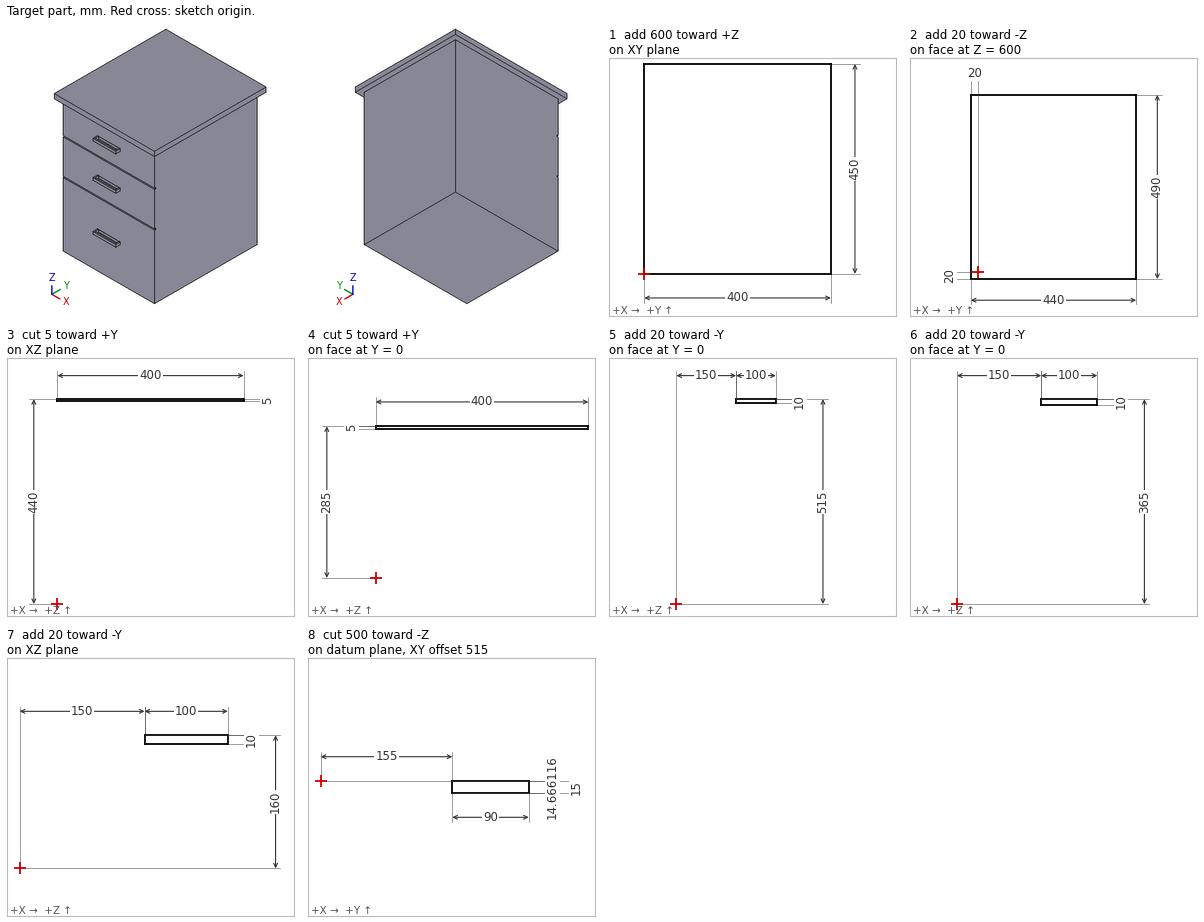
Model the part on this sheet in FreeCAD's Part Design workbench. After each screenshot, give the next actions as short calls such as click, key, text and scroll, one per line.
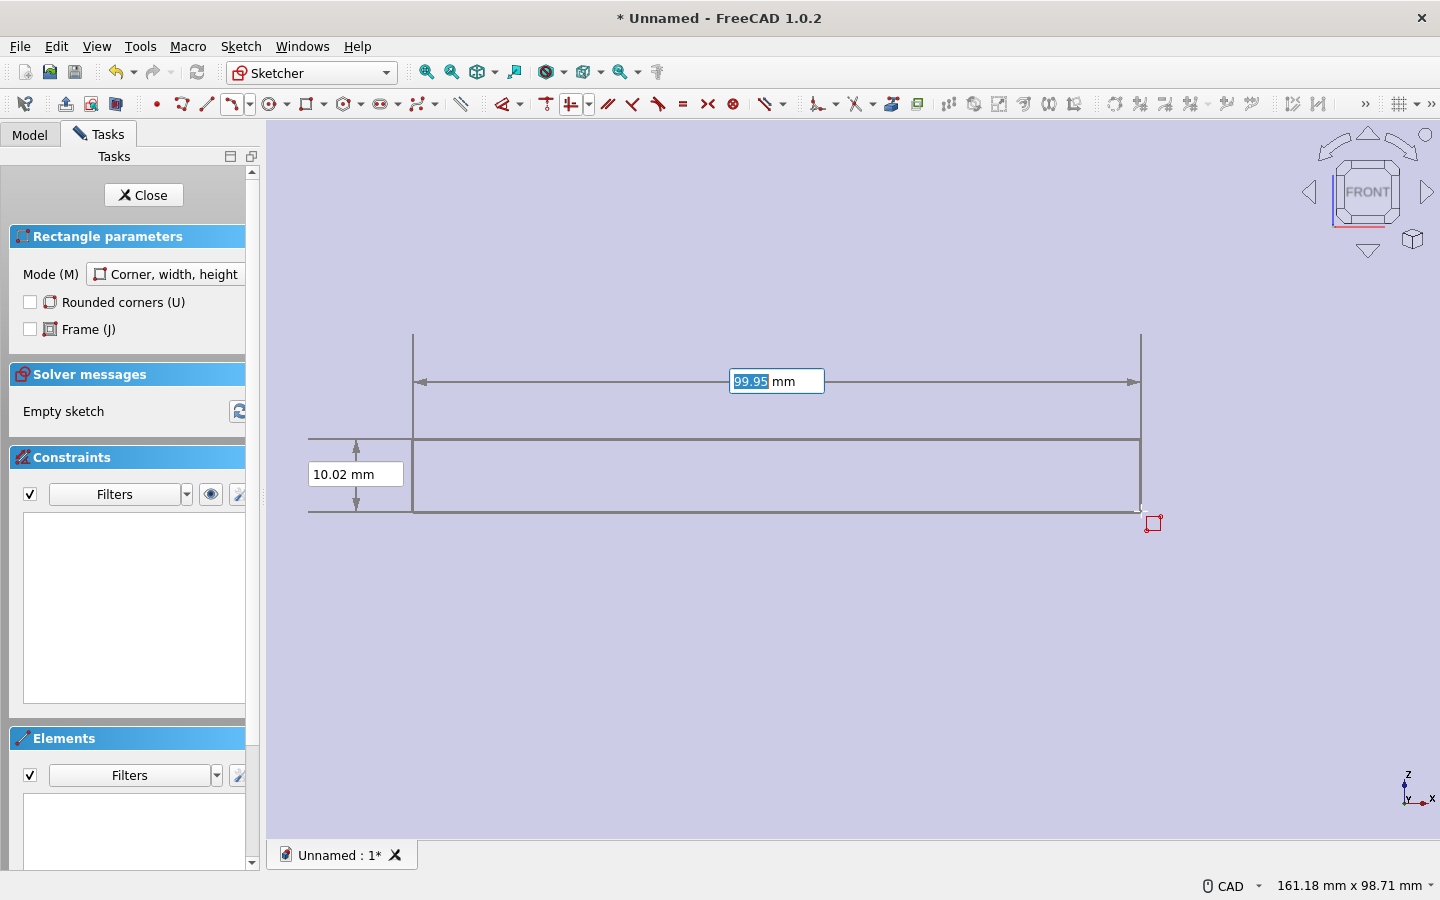
text(100)
key(Tab)
text(10)
key(Return)
key(Escape)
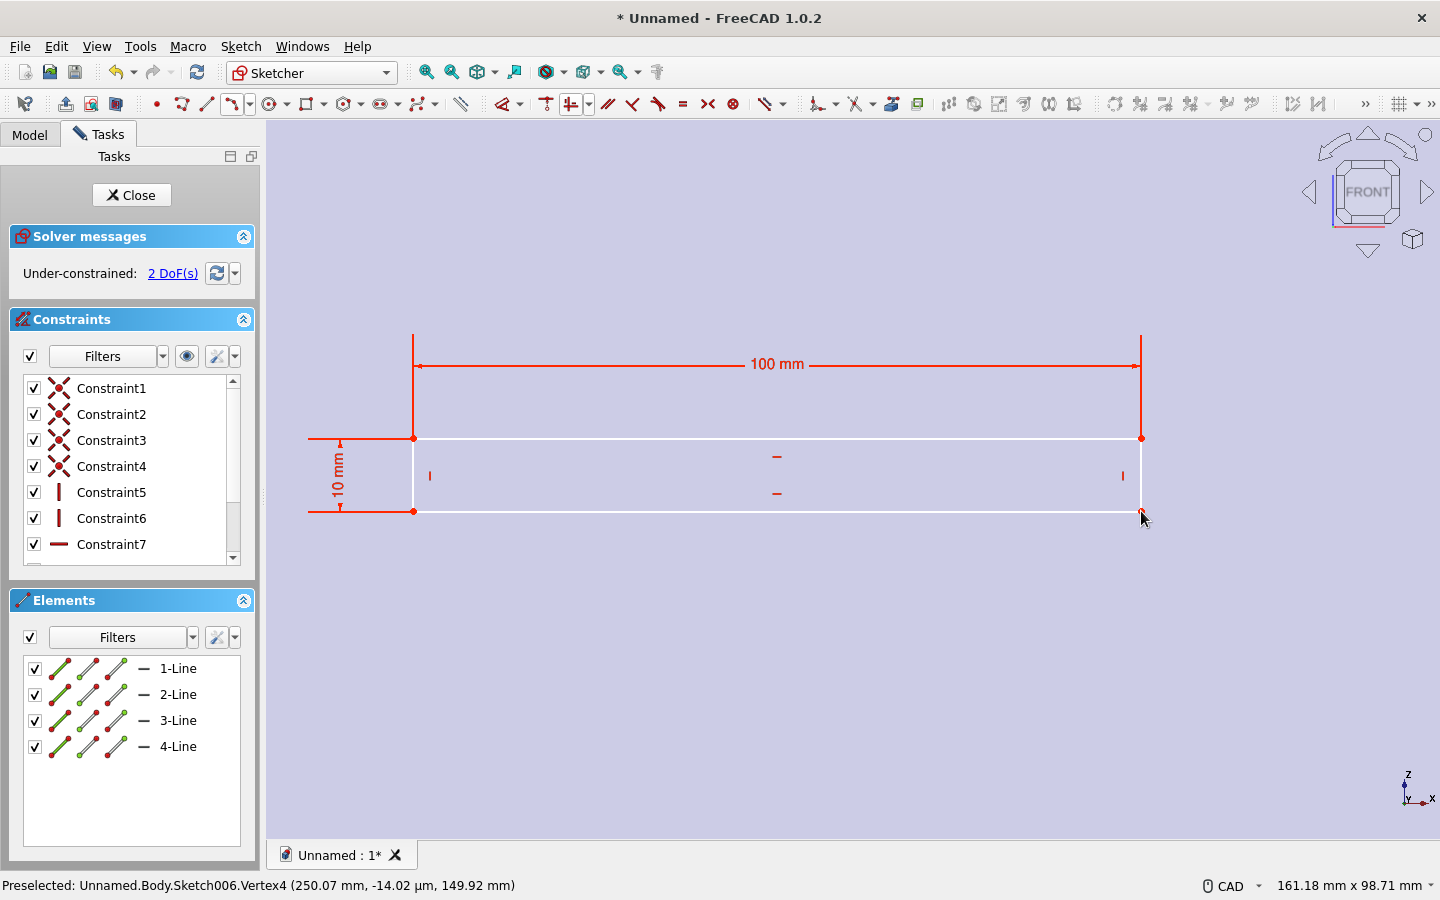
key(d)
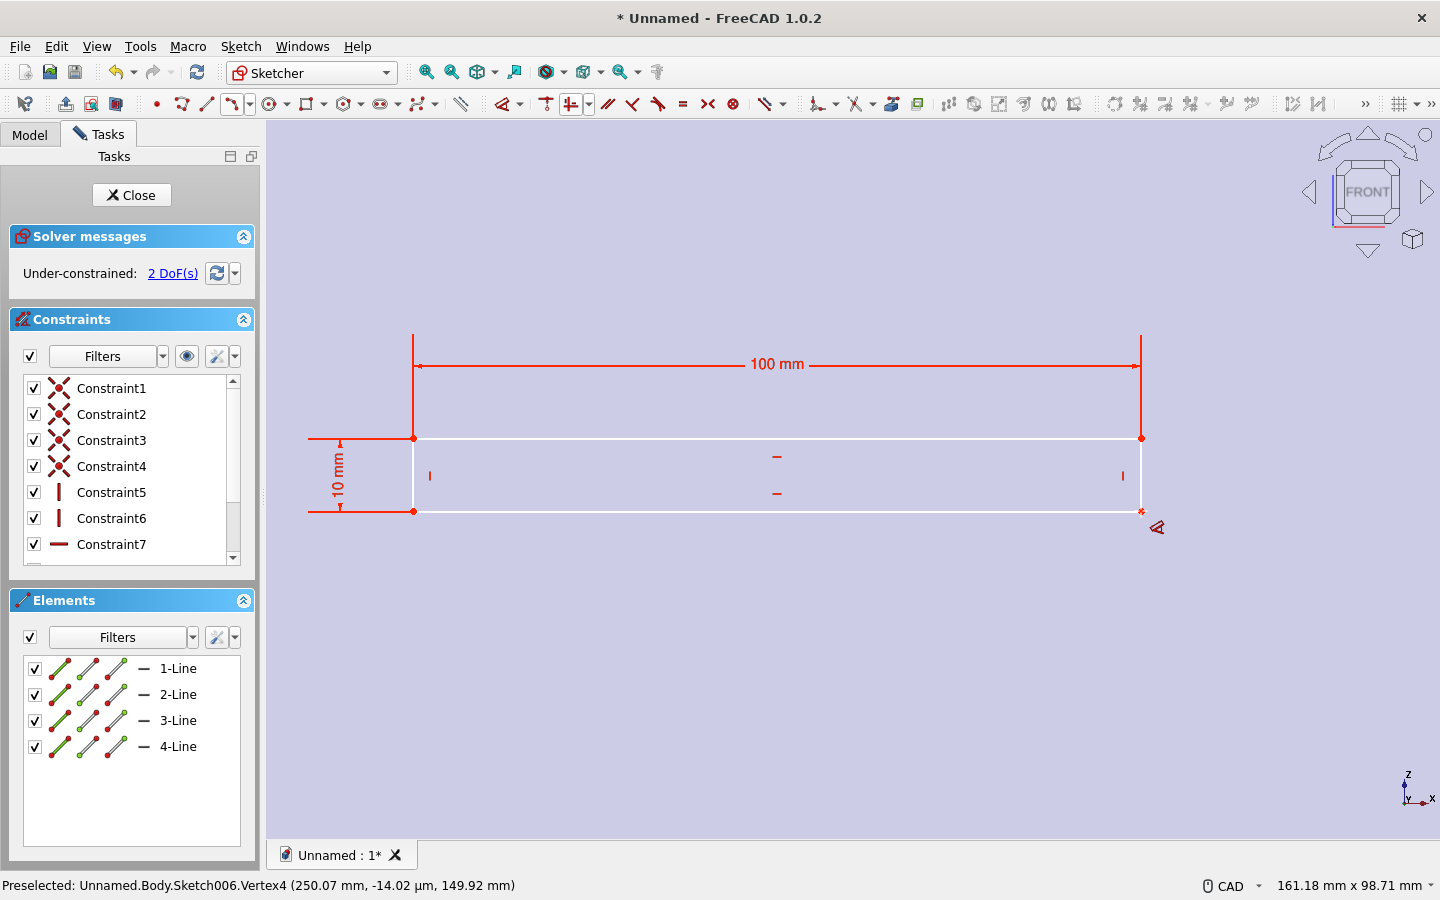
click(413, 439)
click(354, 405)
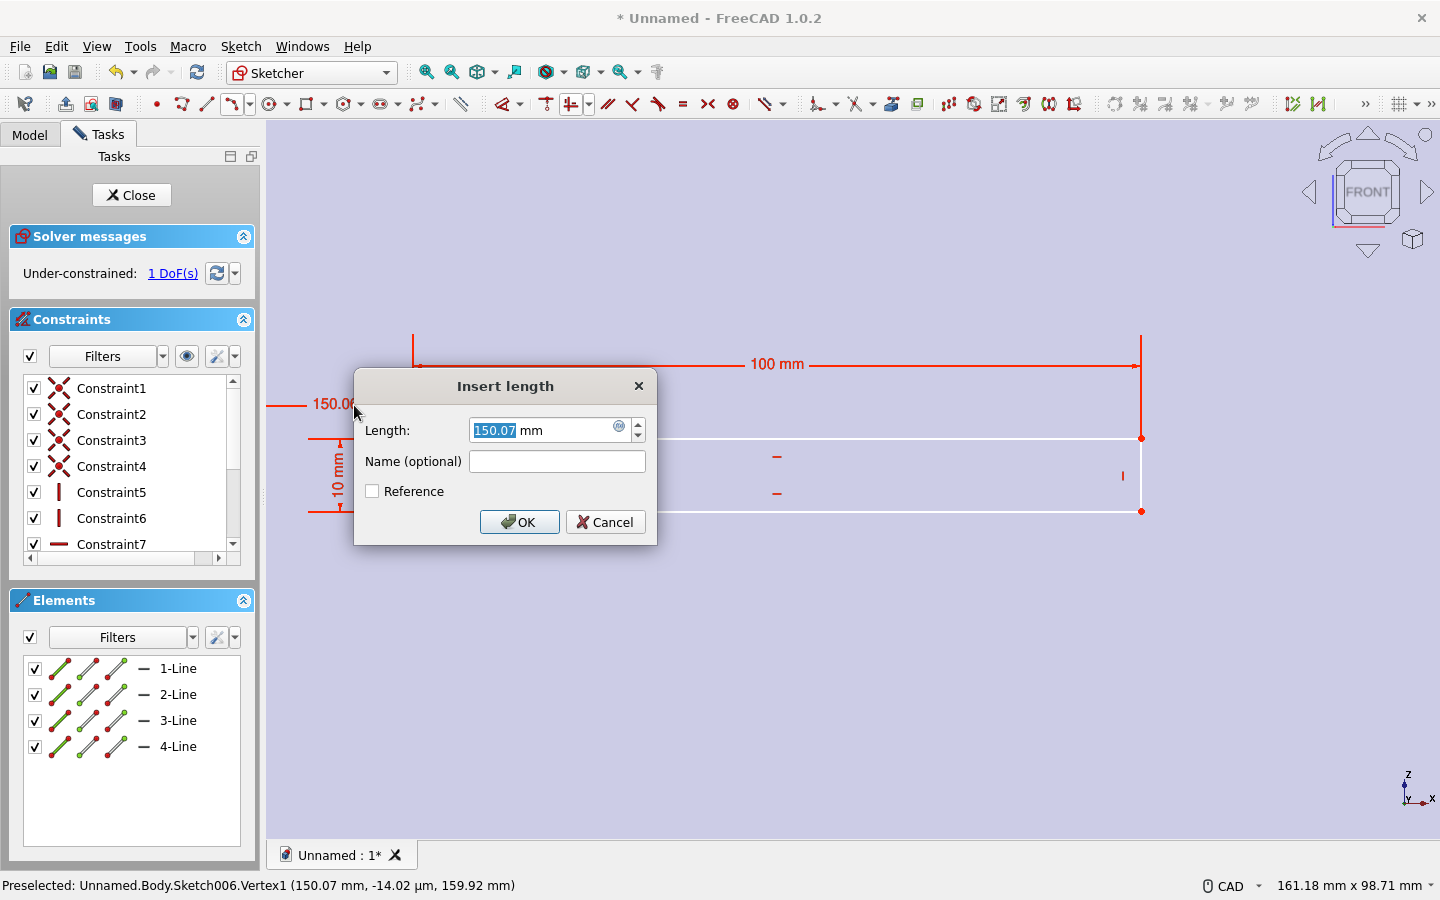
text(150)
key(Return)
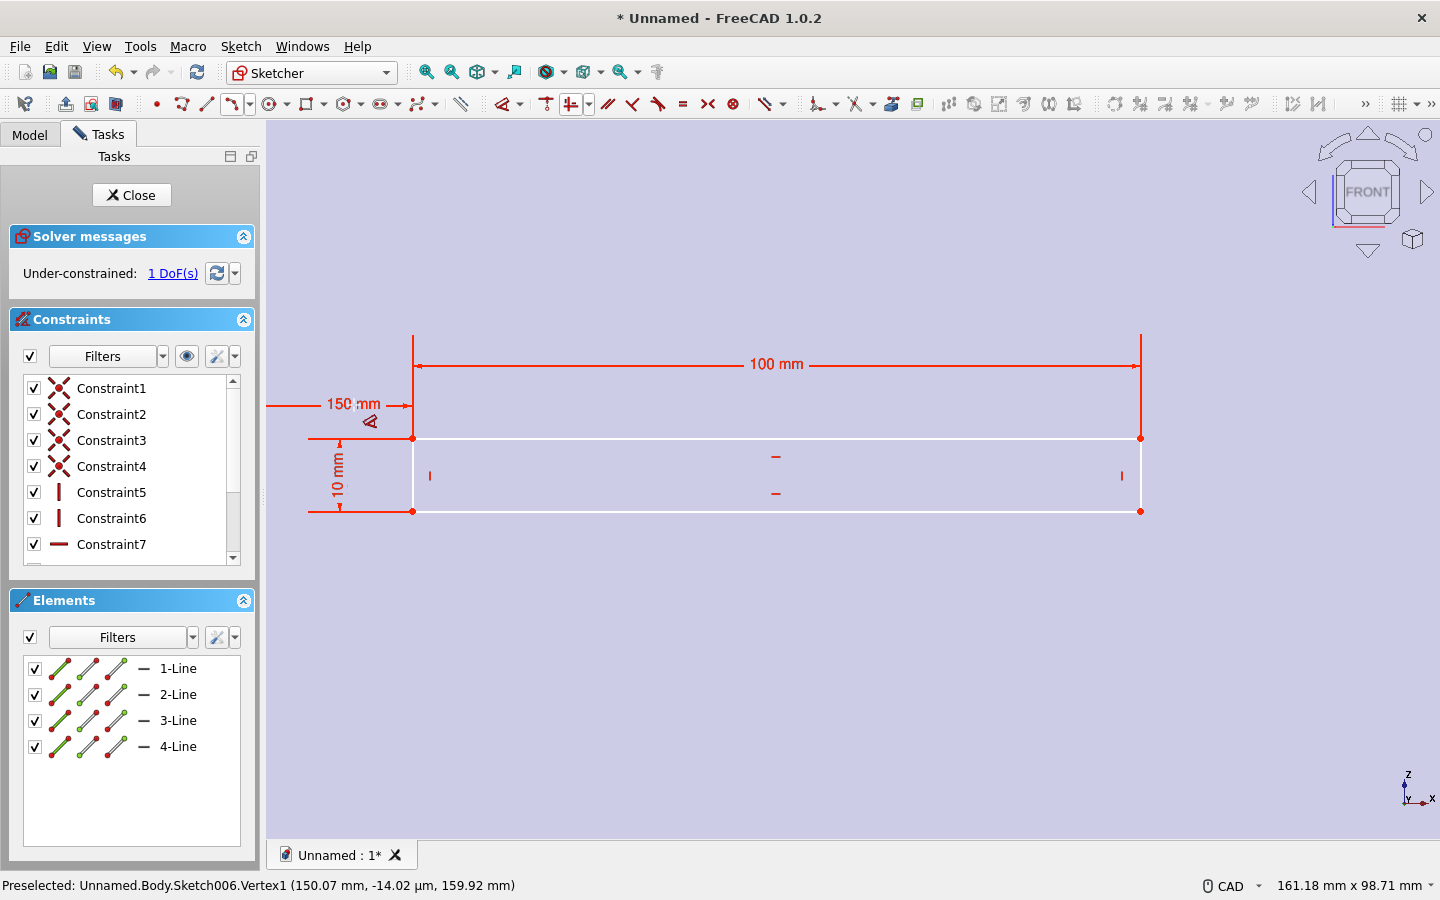
click(413, 439)
click(447, 625)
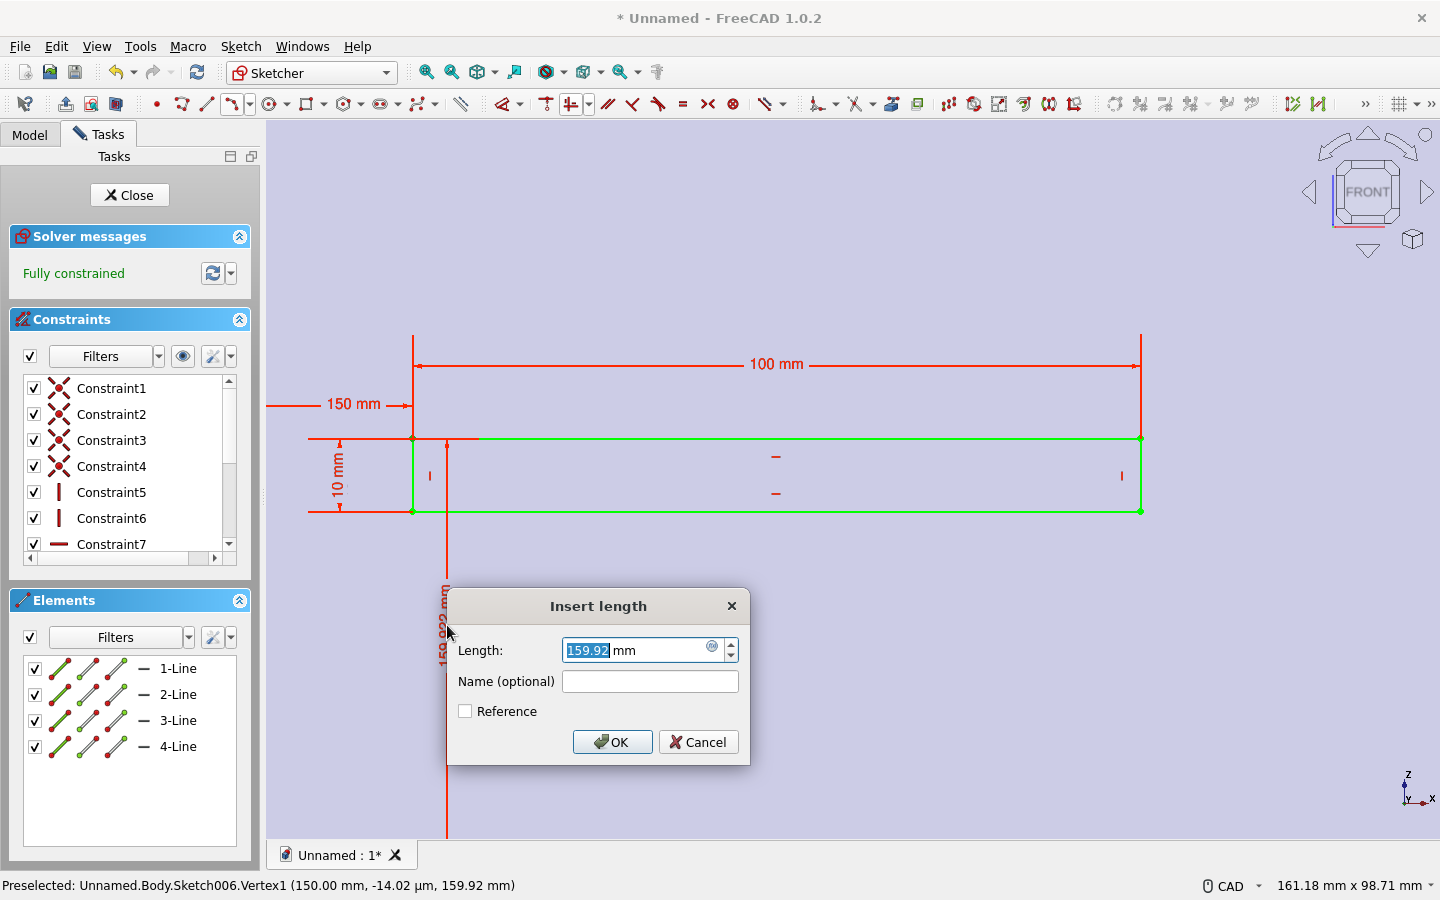
text(160)
key(Return)
key(Escape)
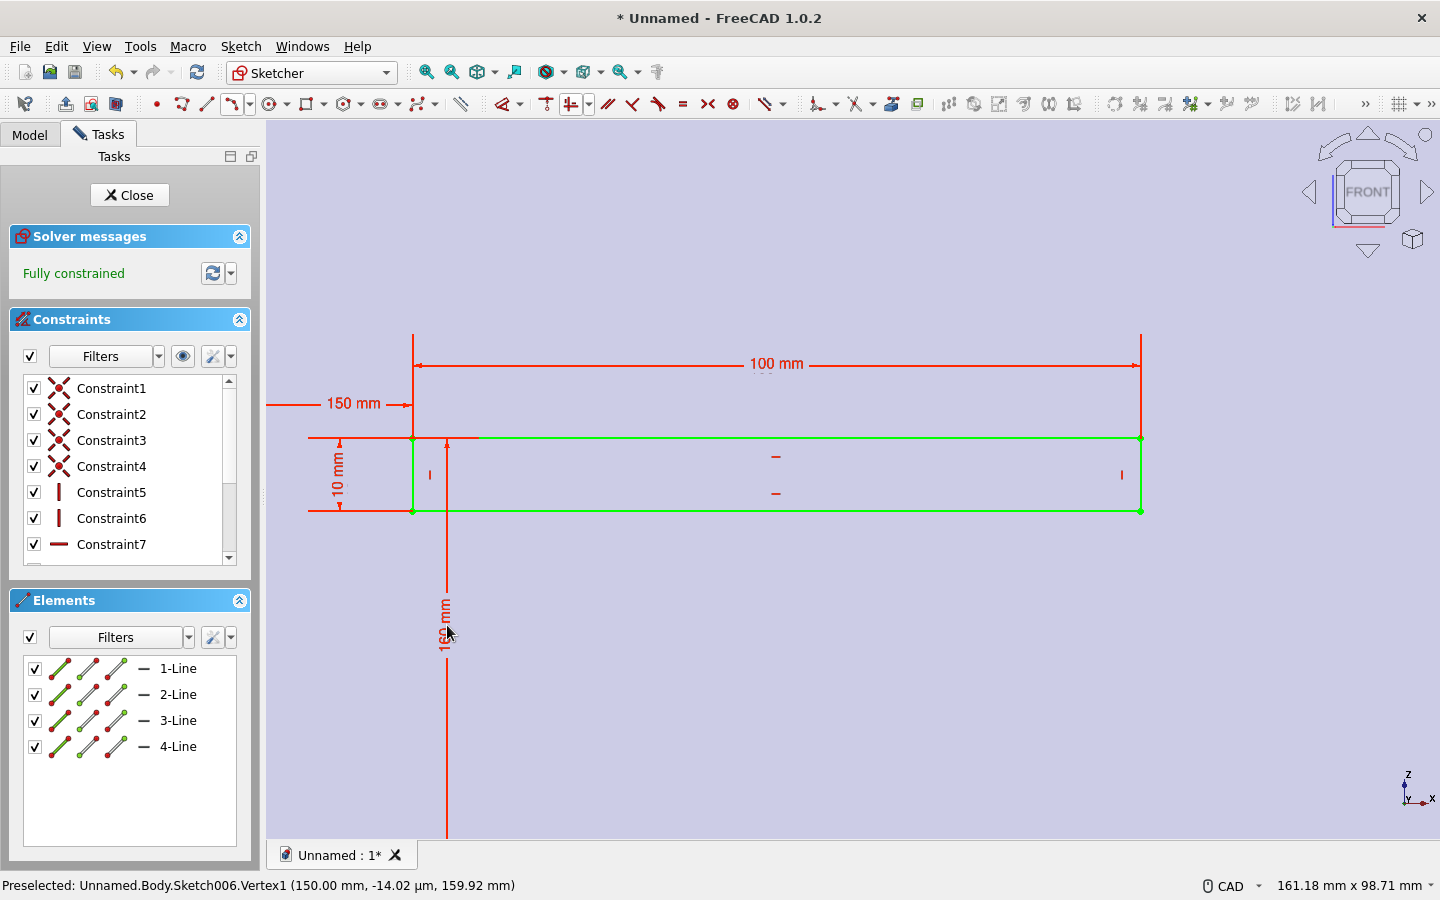
click(130, 195)